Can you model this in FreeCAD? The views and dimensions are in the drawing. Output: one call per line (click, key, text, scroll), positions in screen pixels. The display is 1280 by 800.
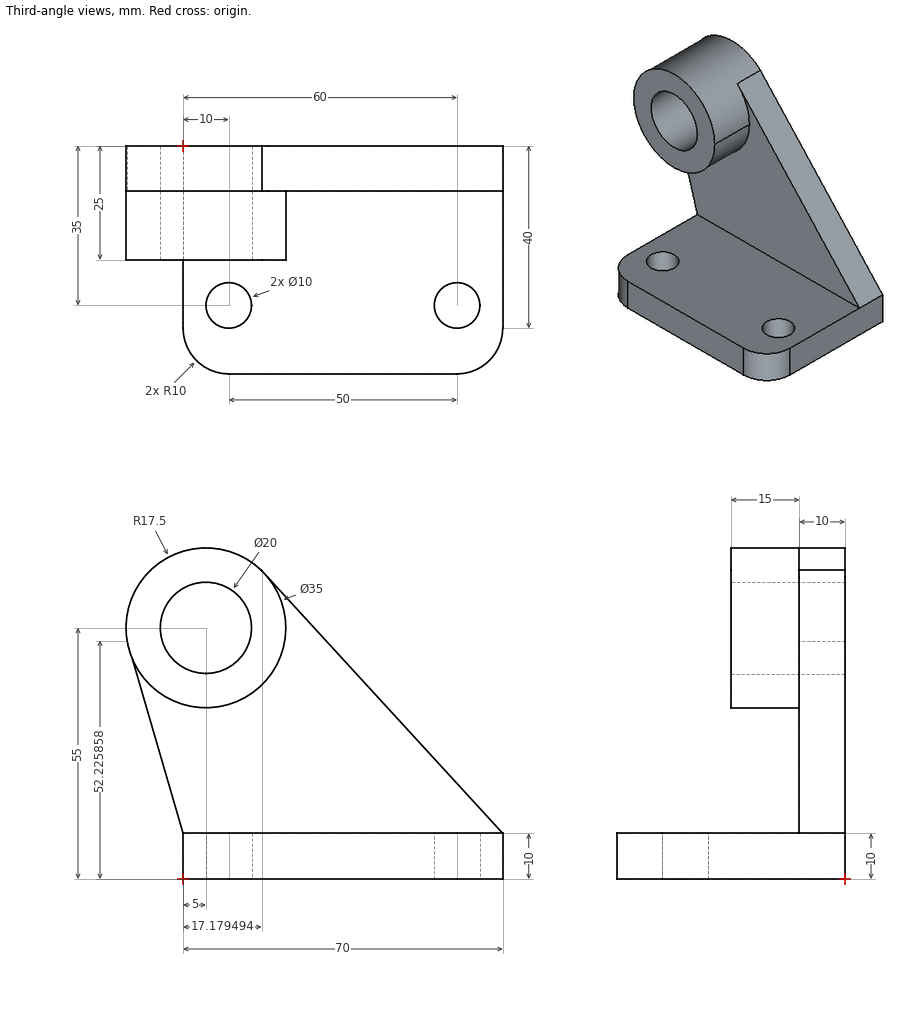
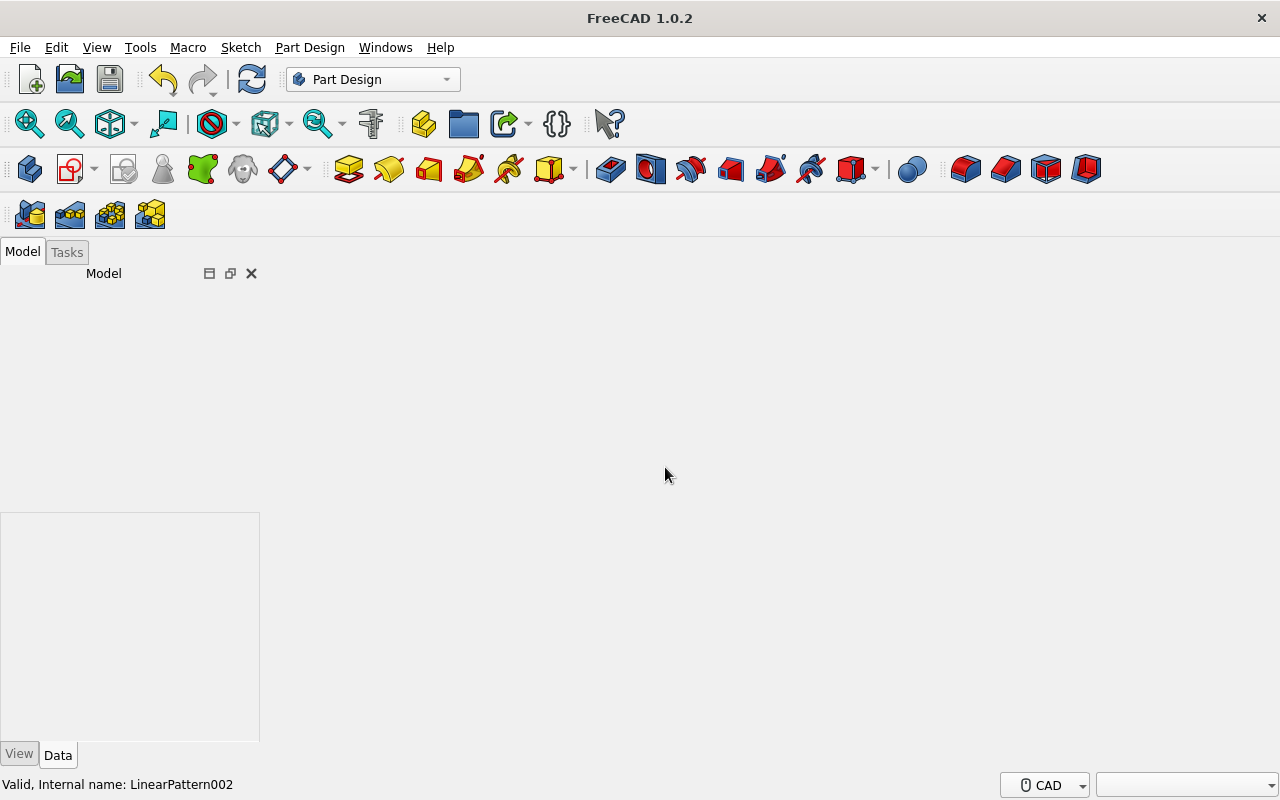
key(ctrl+n)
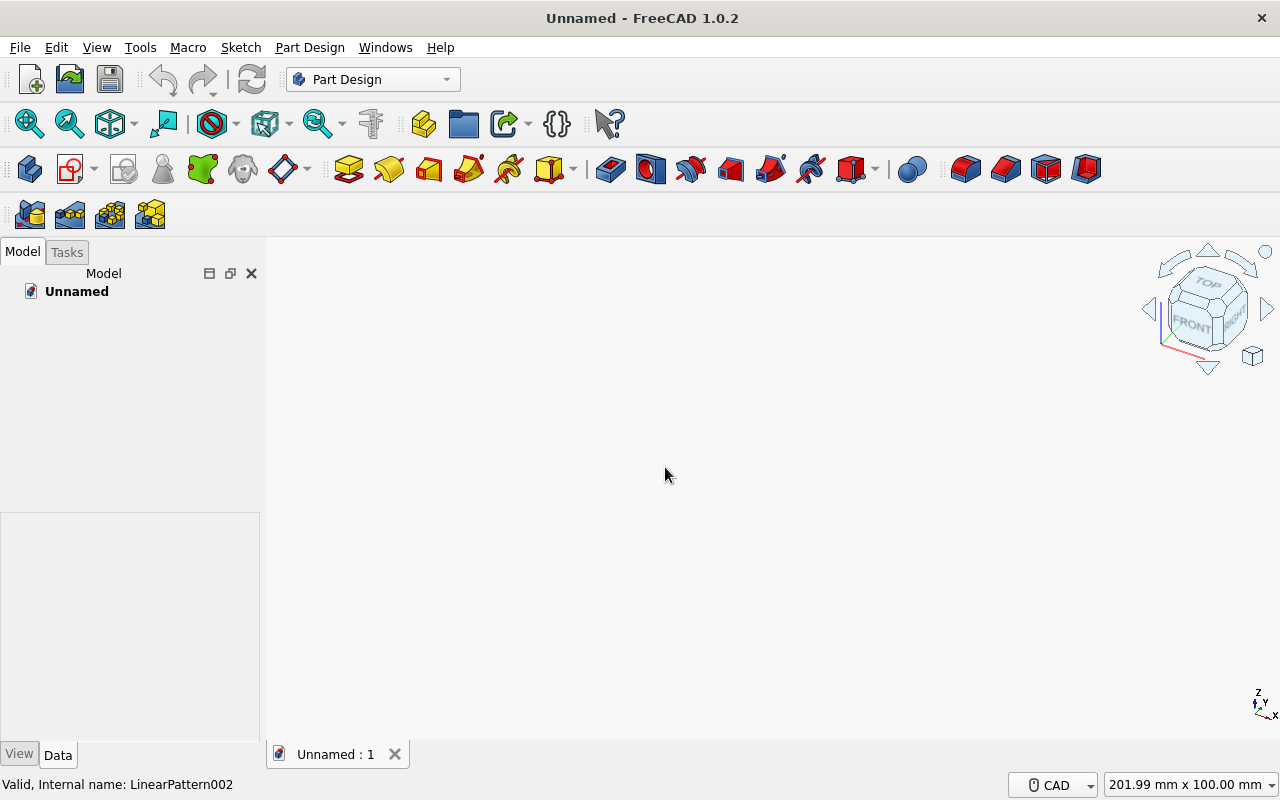
click(70, 170)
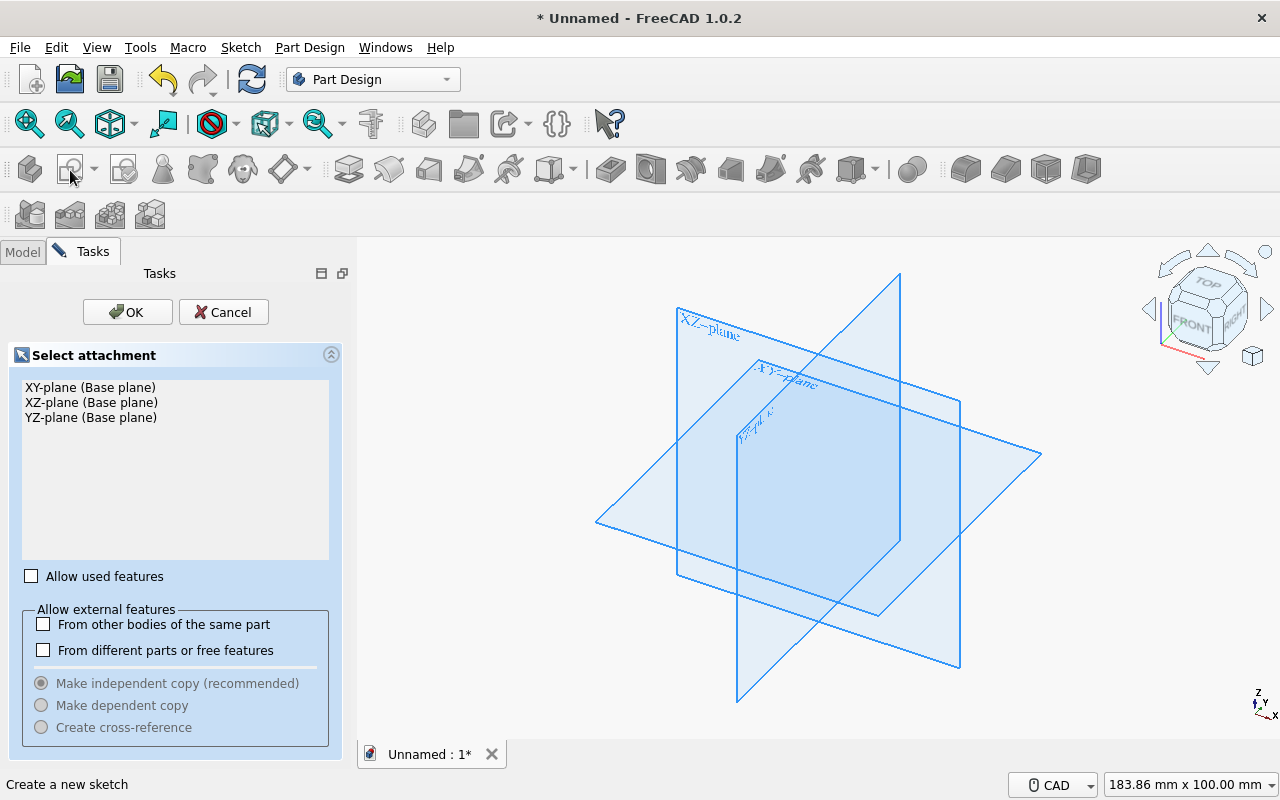
click(82, 388)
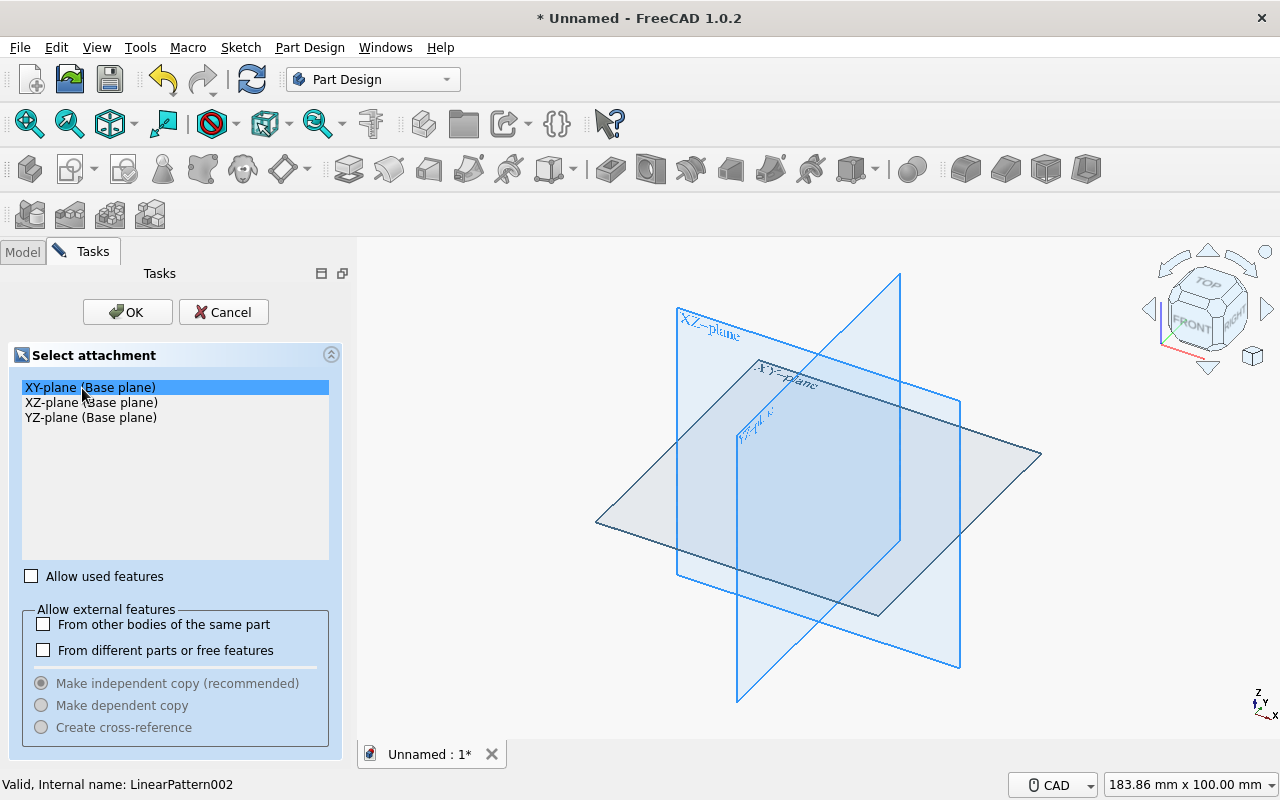
click(128, 312)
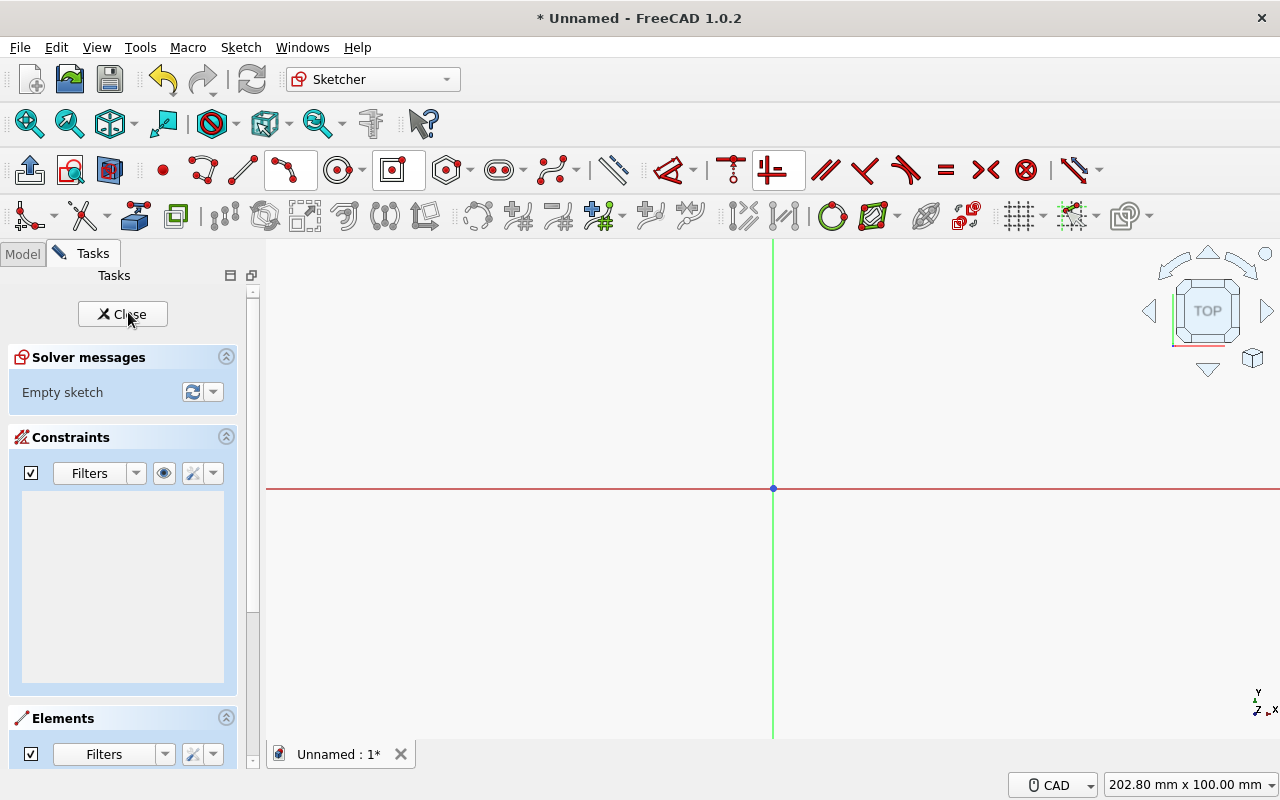
scroll(294, 267, down, 1)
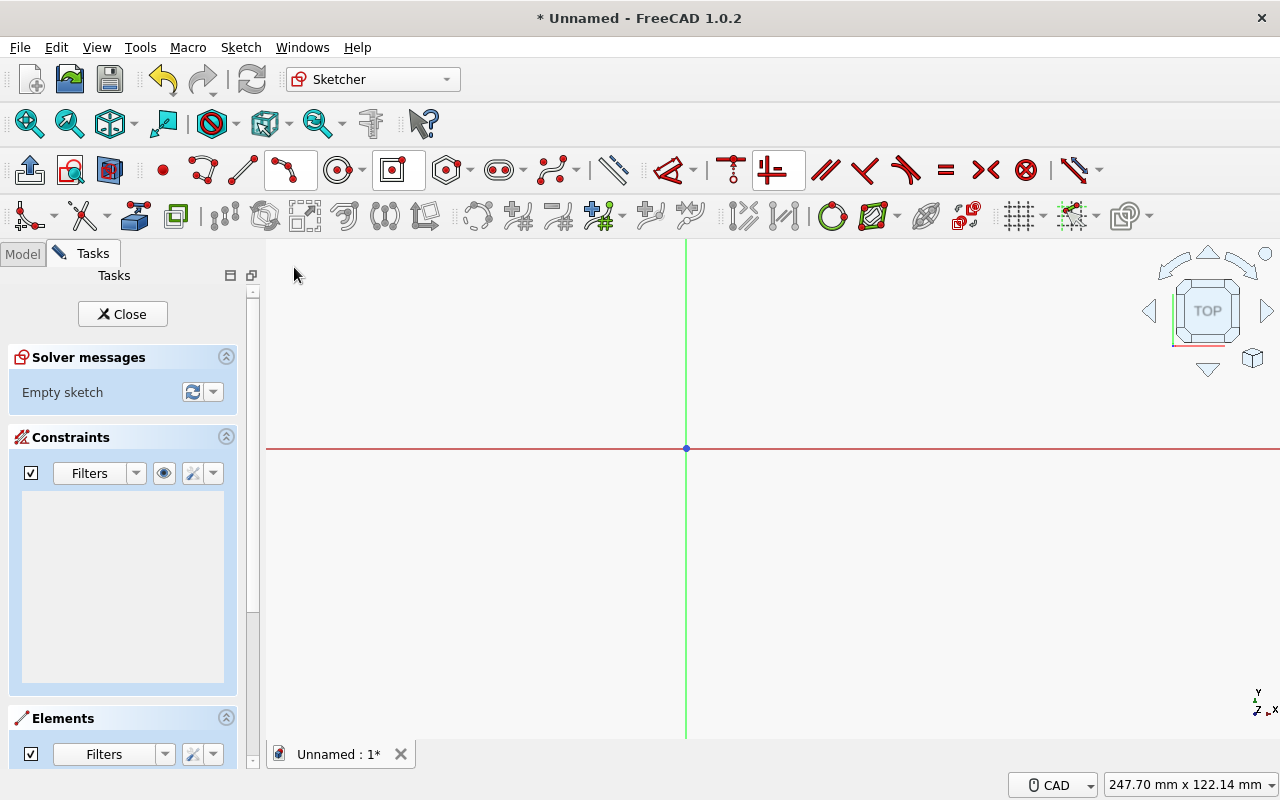
scroll(1084, 677, up, 2)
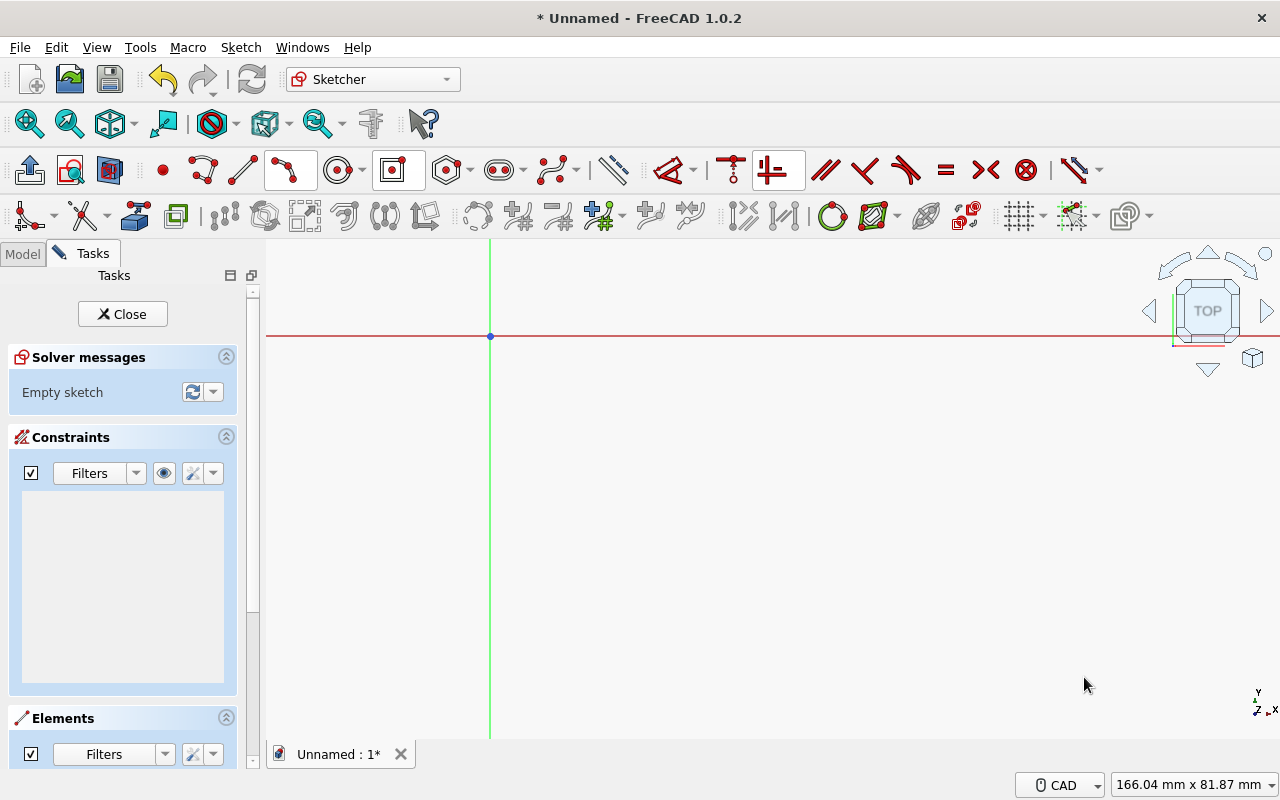
click(244, 170)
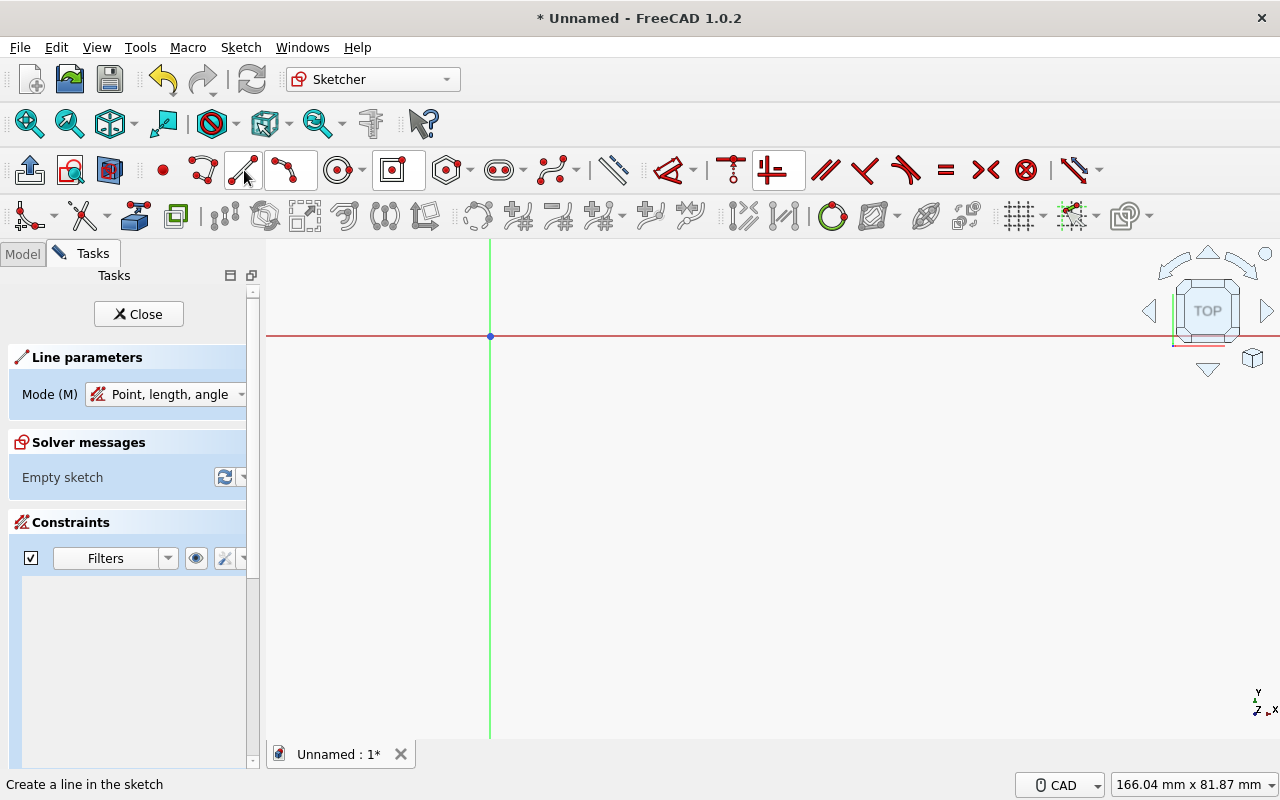
click(551, 641)
click(857, 641)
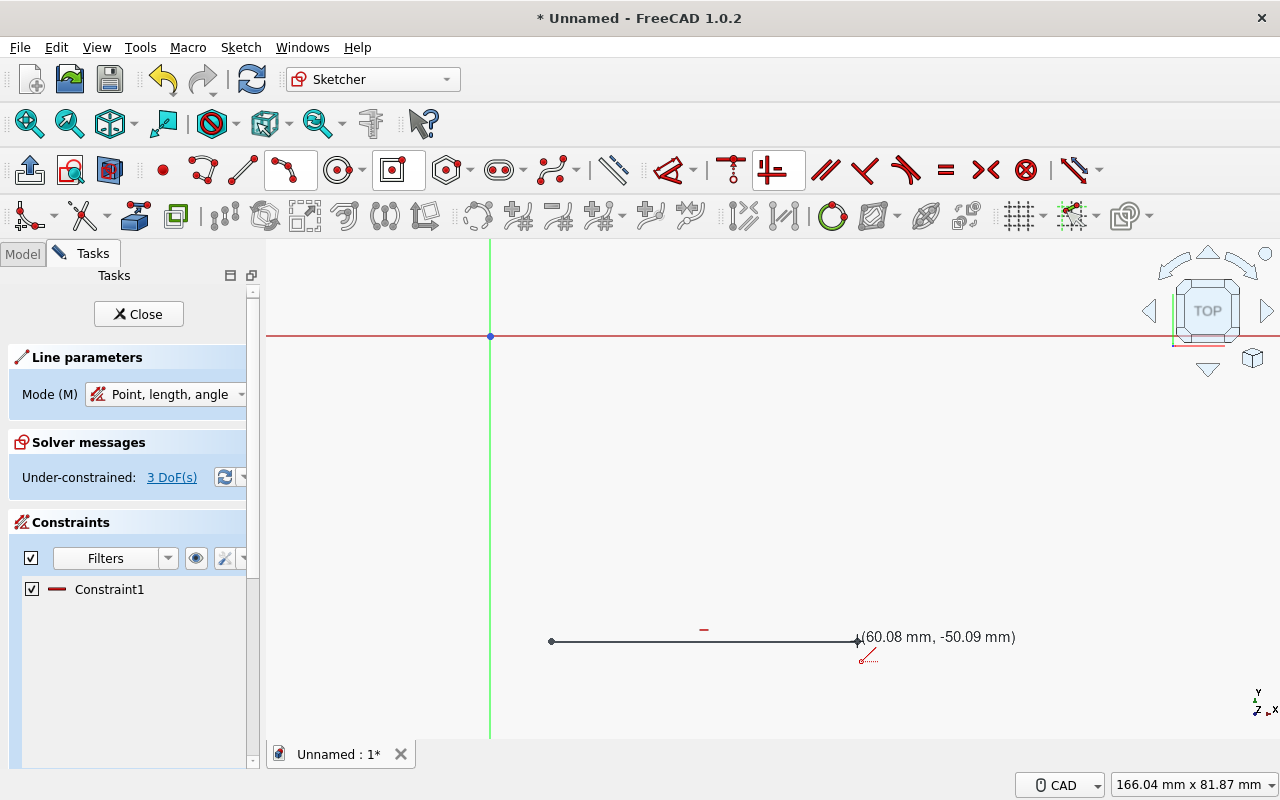
click(204, 170)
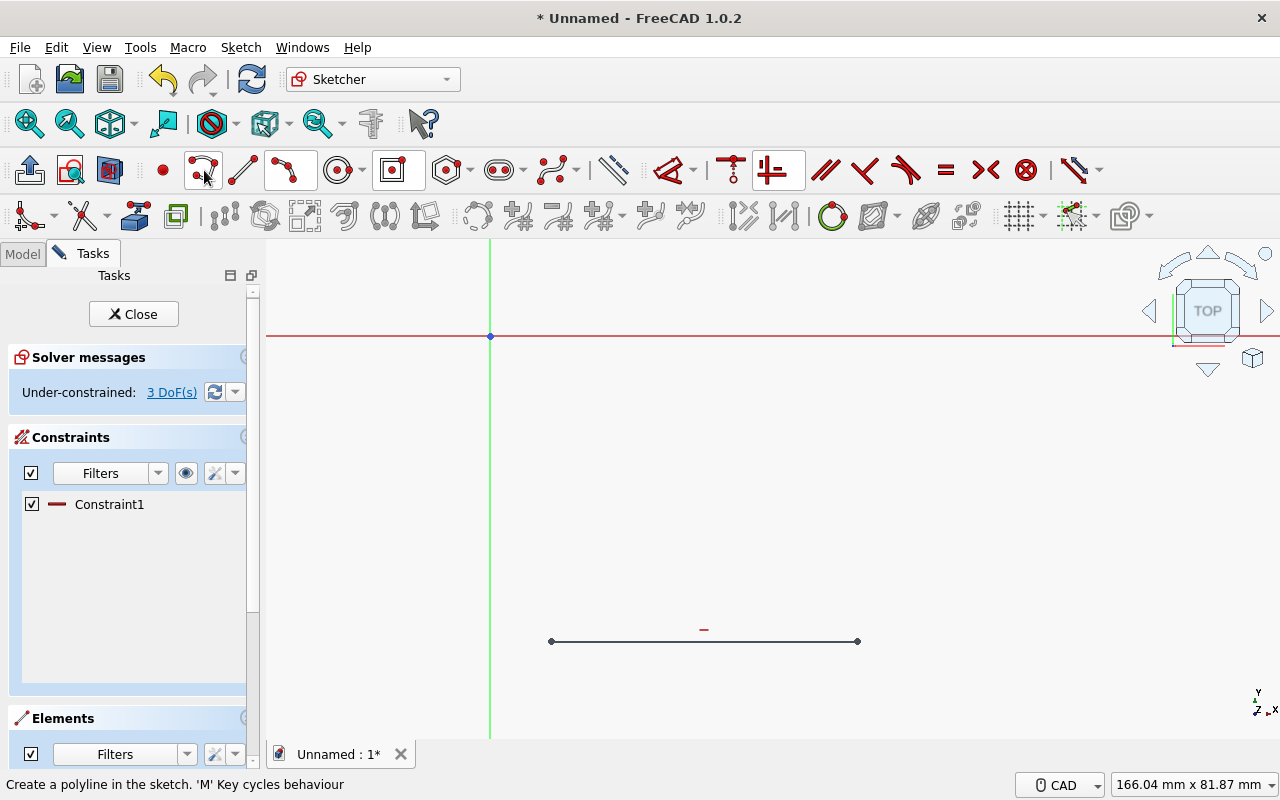
click(918, 580)
click(918, 336)
click(490, 336)
click(499, 580)
right_click(499, 580)